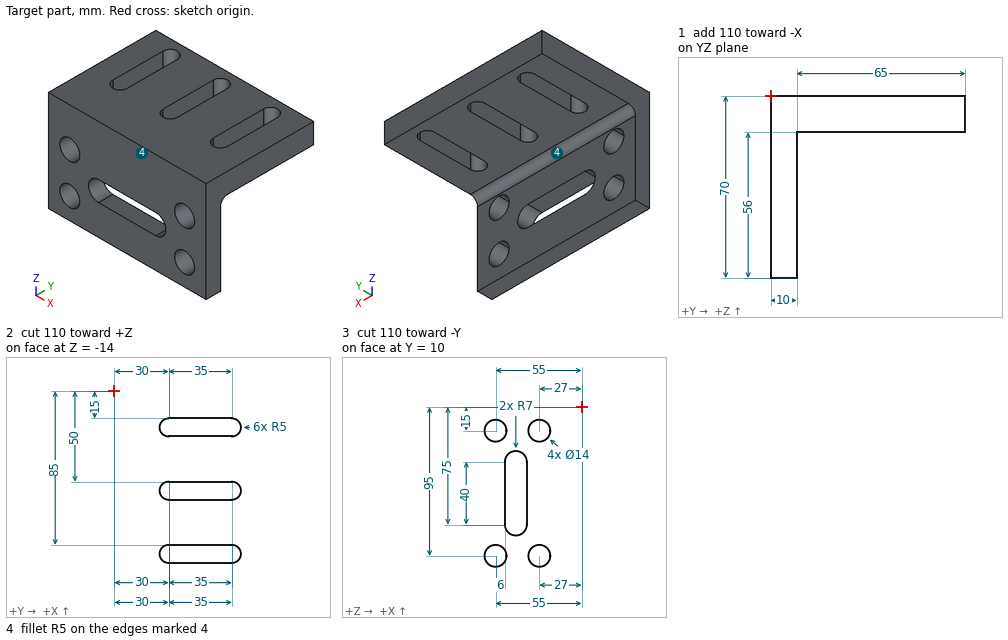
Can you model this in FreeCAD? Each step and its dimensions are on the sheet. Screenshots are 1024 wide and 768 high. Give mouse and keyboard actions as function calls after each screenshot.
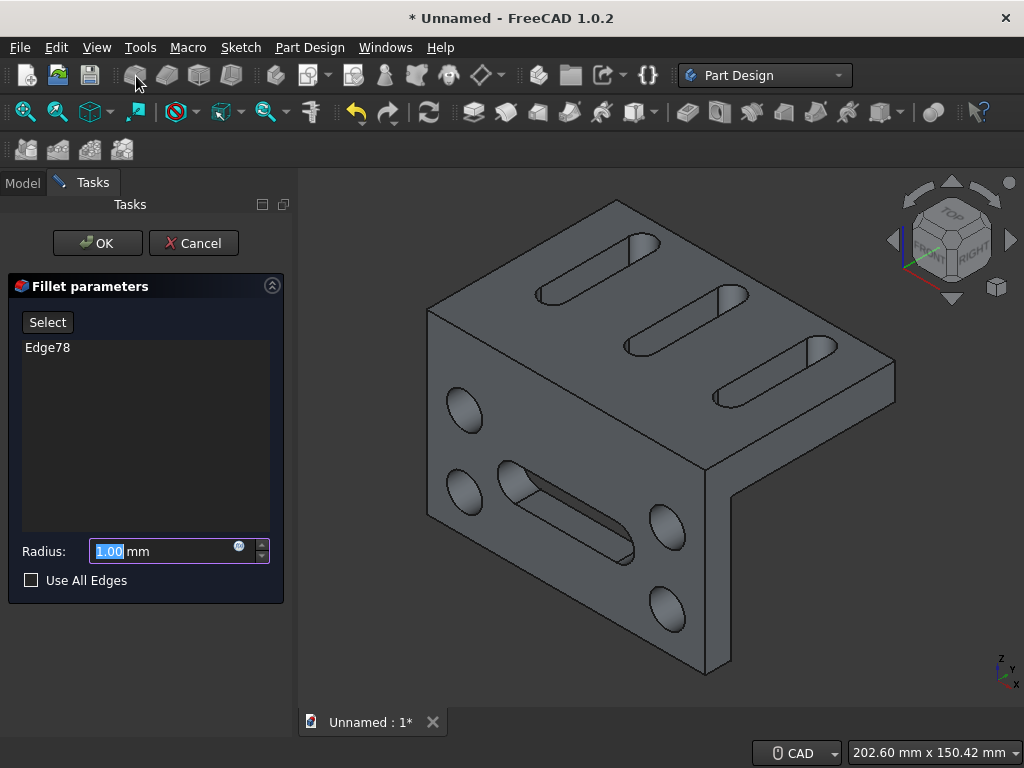
text(5)
key(Tab)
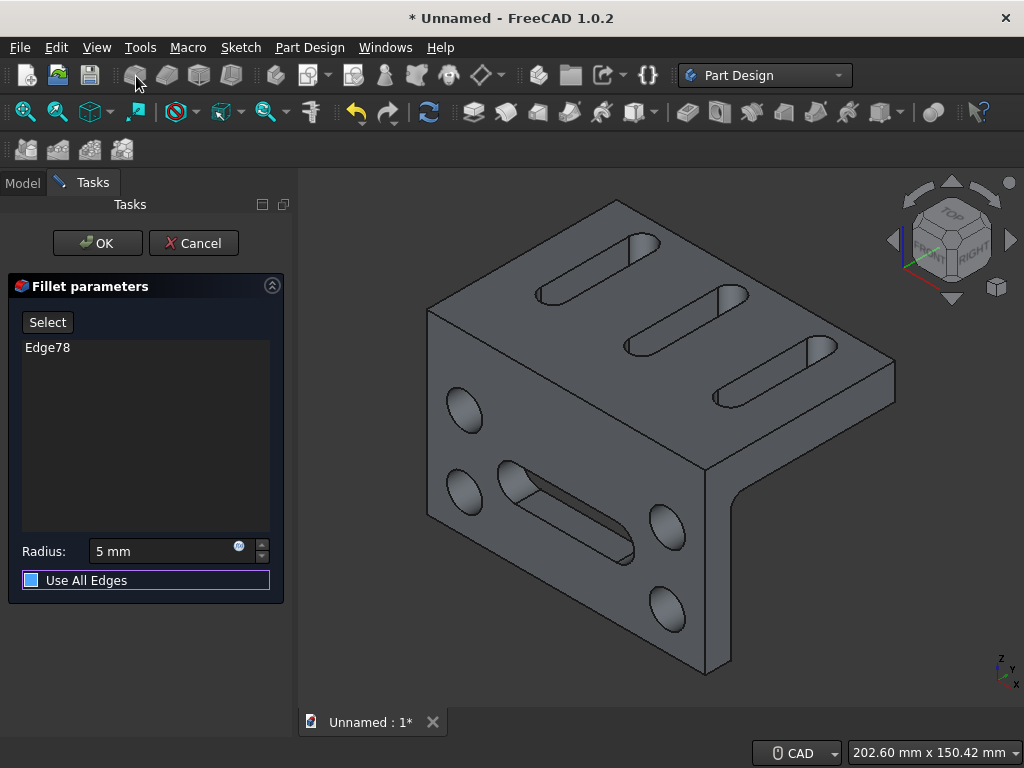
click(98, 243)